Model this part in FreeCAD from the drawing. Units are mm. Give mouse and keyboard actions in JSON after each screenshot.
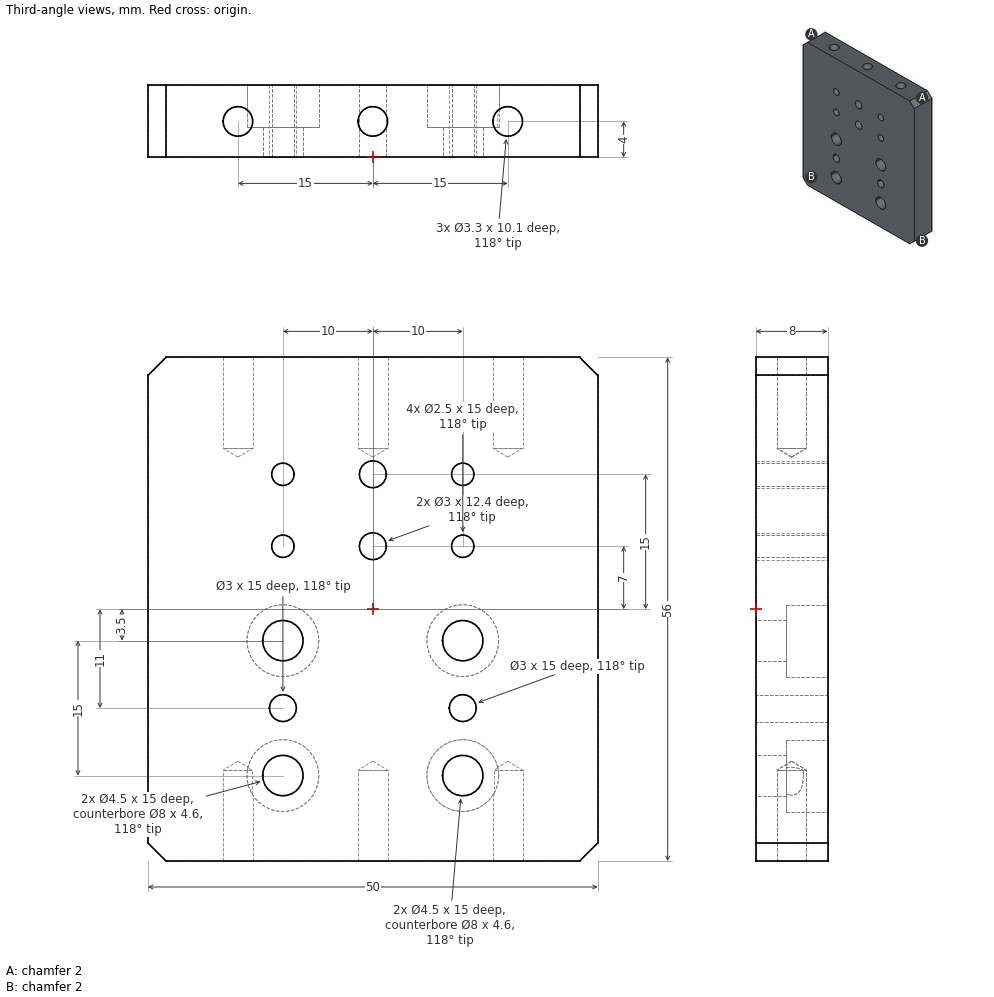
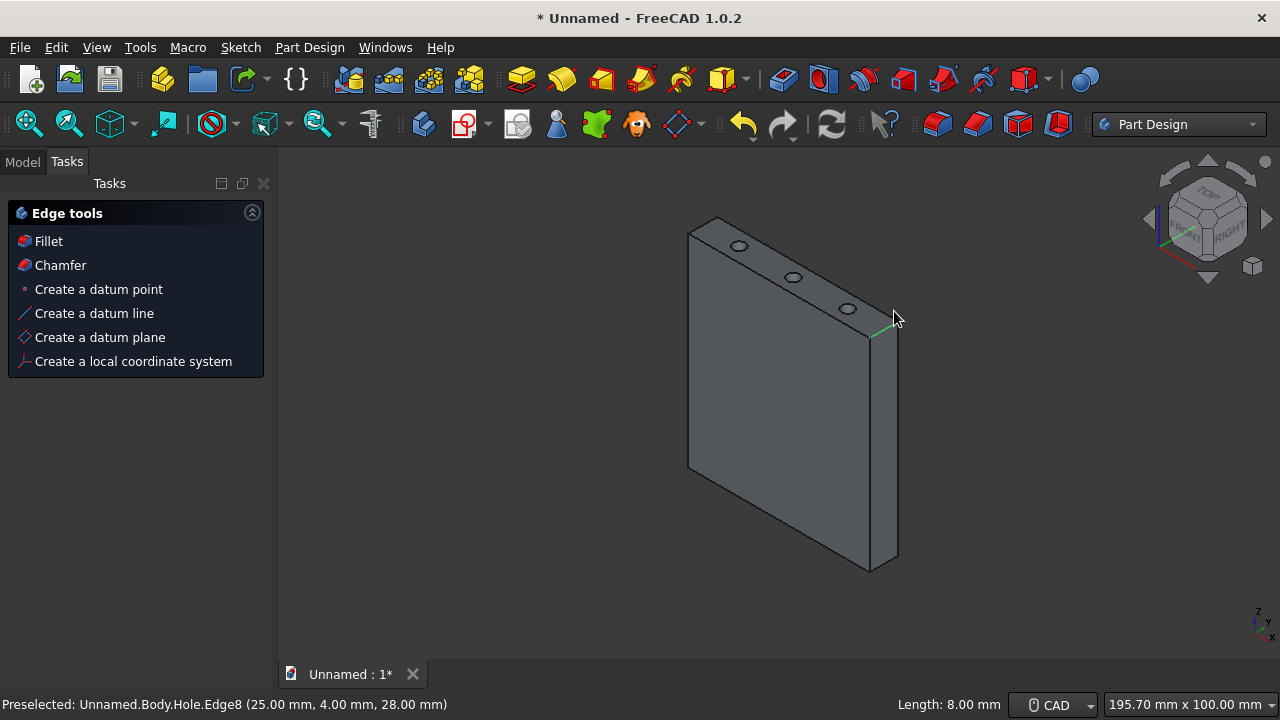
{"action": "key", "text": "2"}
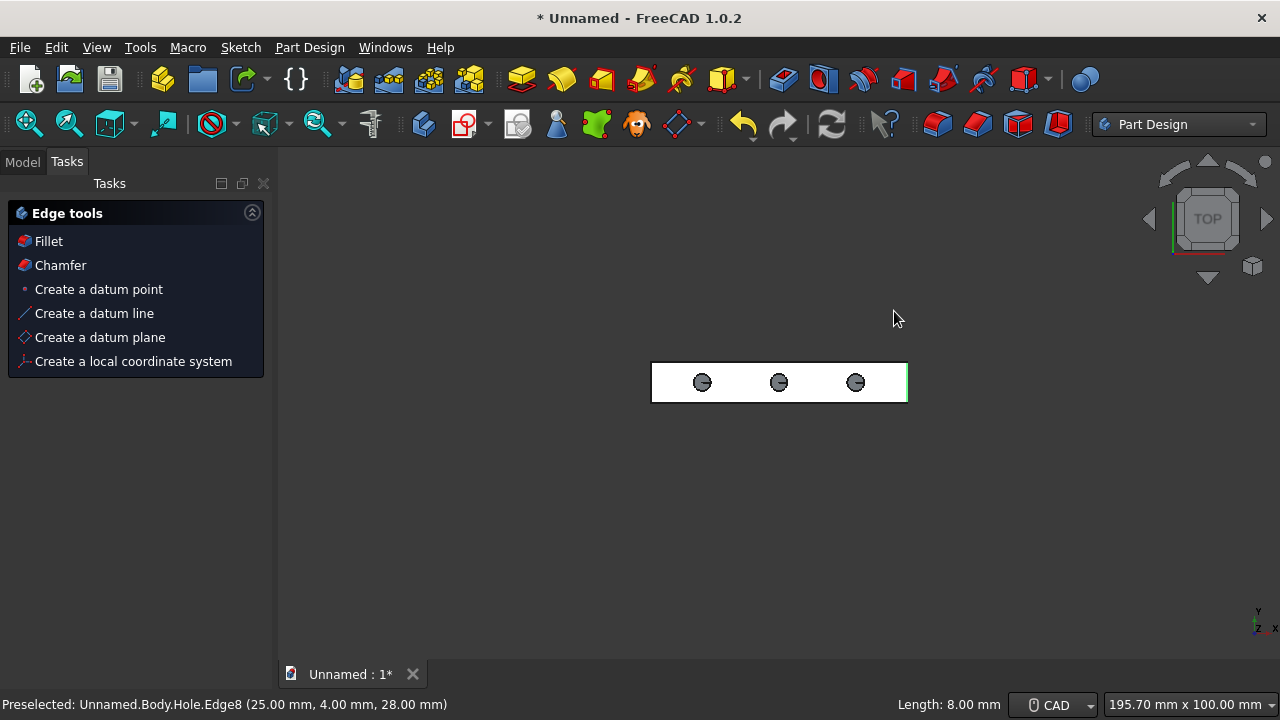
{"action": "left_click", "coordinate": [30, 124]}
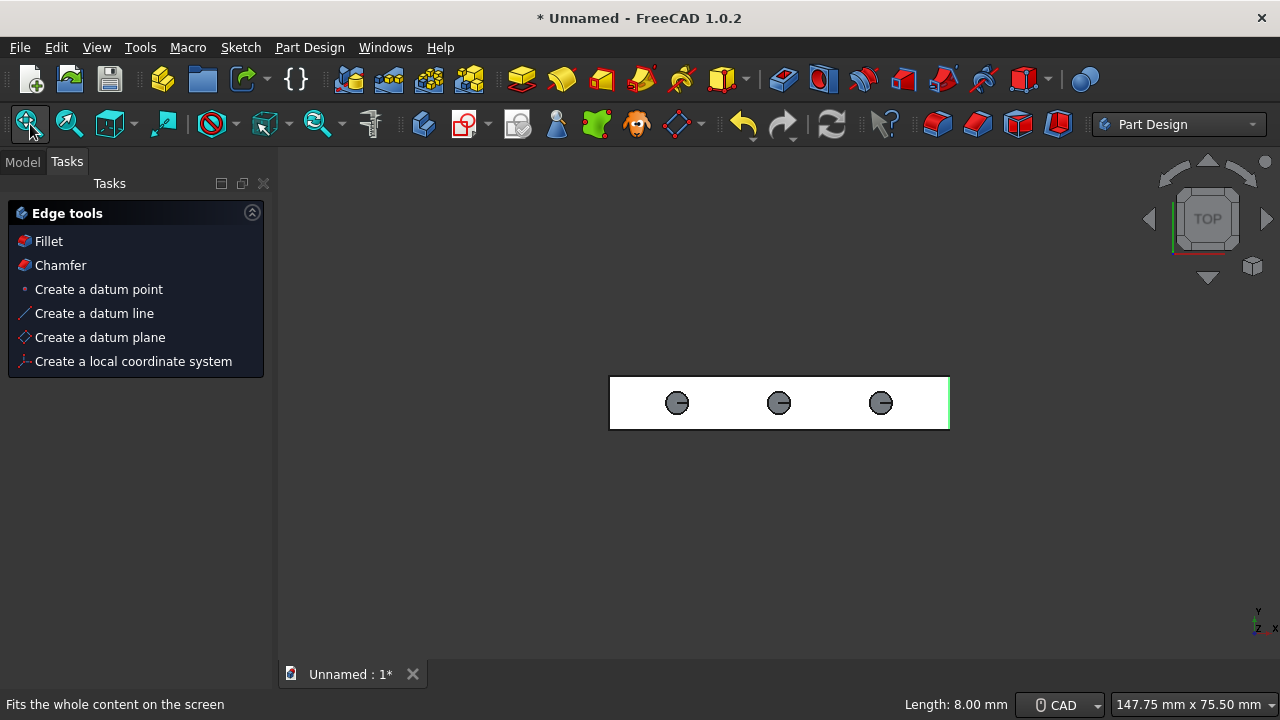
{"action": "left_click", "coordinate": [609, 402], "text": "ctrl"}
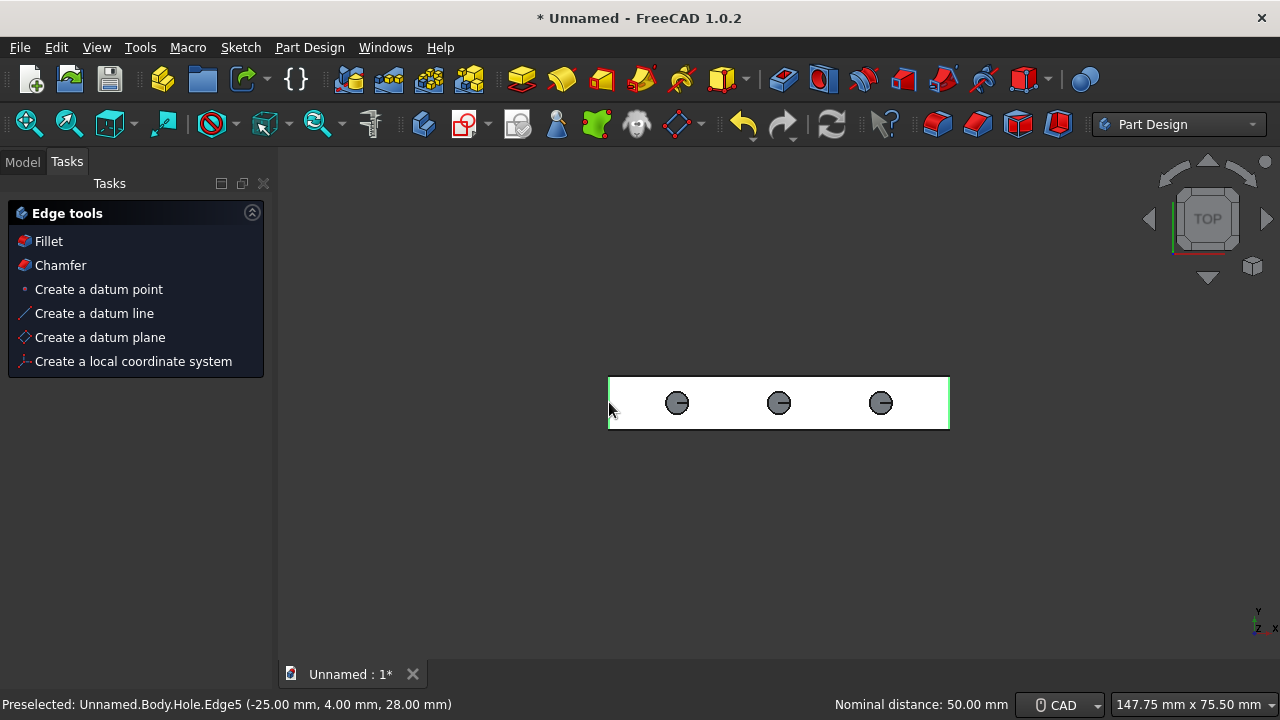
{"action": "left_click", "coordinate": [978, 124]}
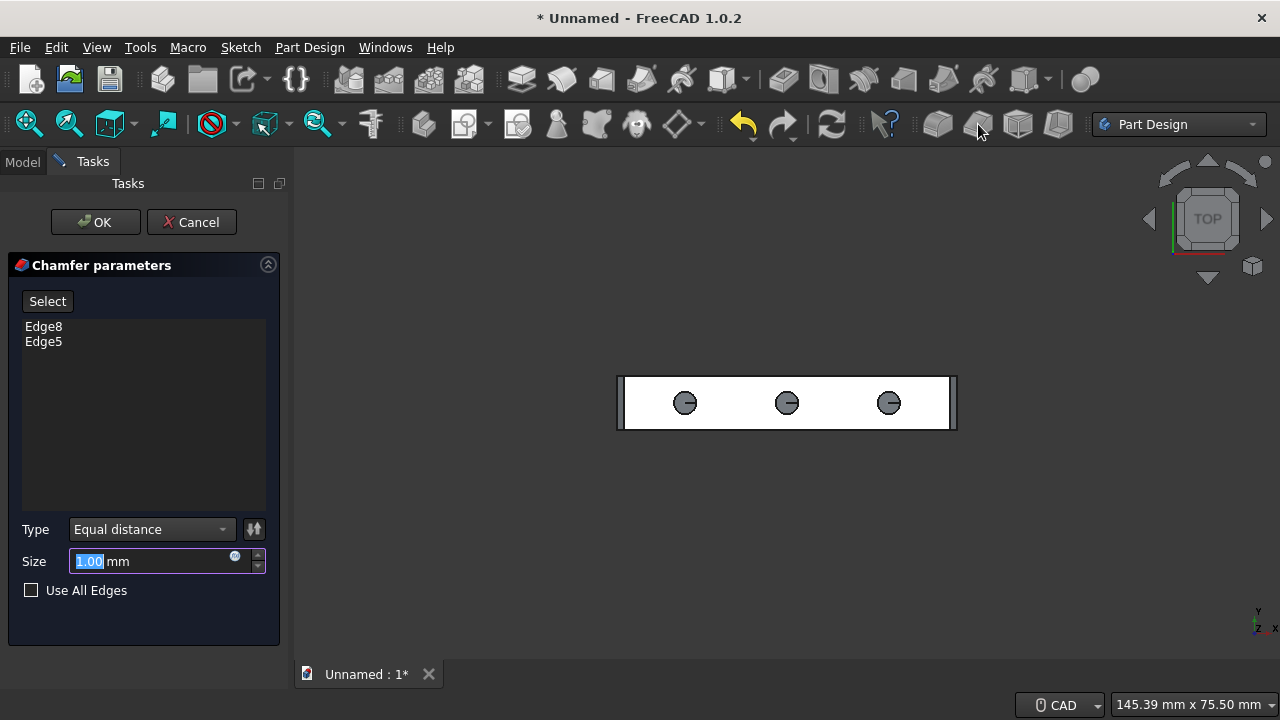
{"action": "type", "text": "2"}
{"action": "key", "text": "Tab"}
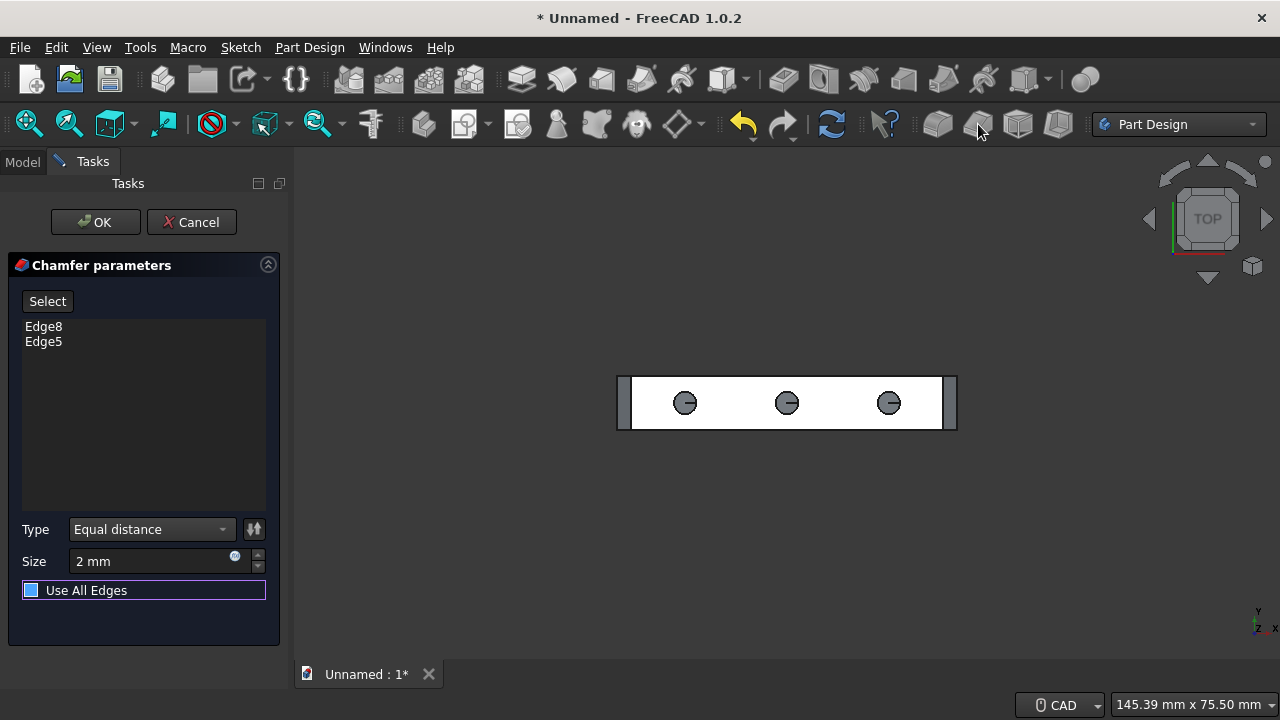
{"action": "left_click", "coordinate": [96, 222]}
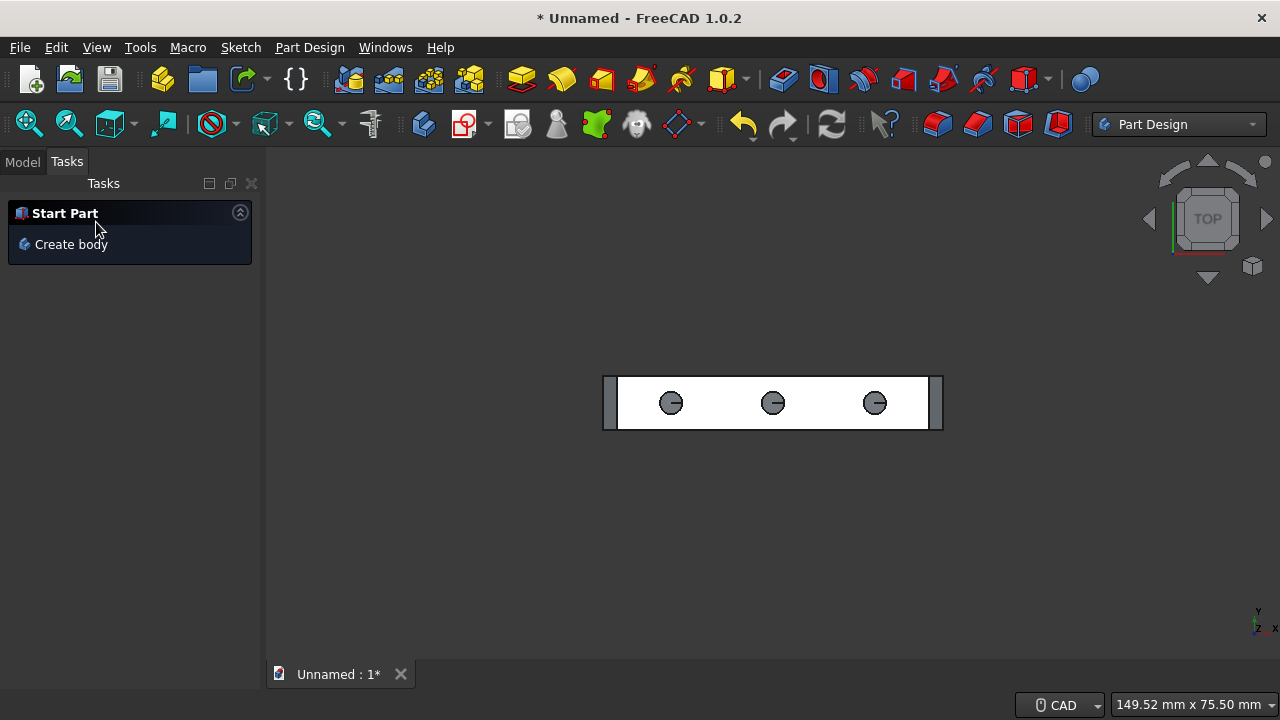
{"action": "left_click", "coordinate": [30, 124]}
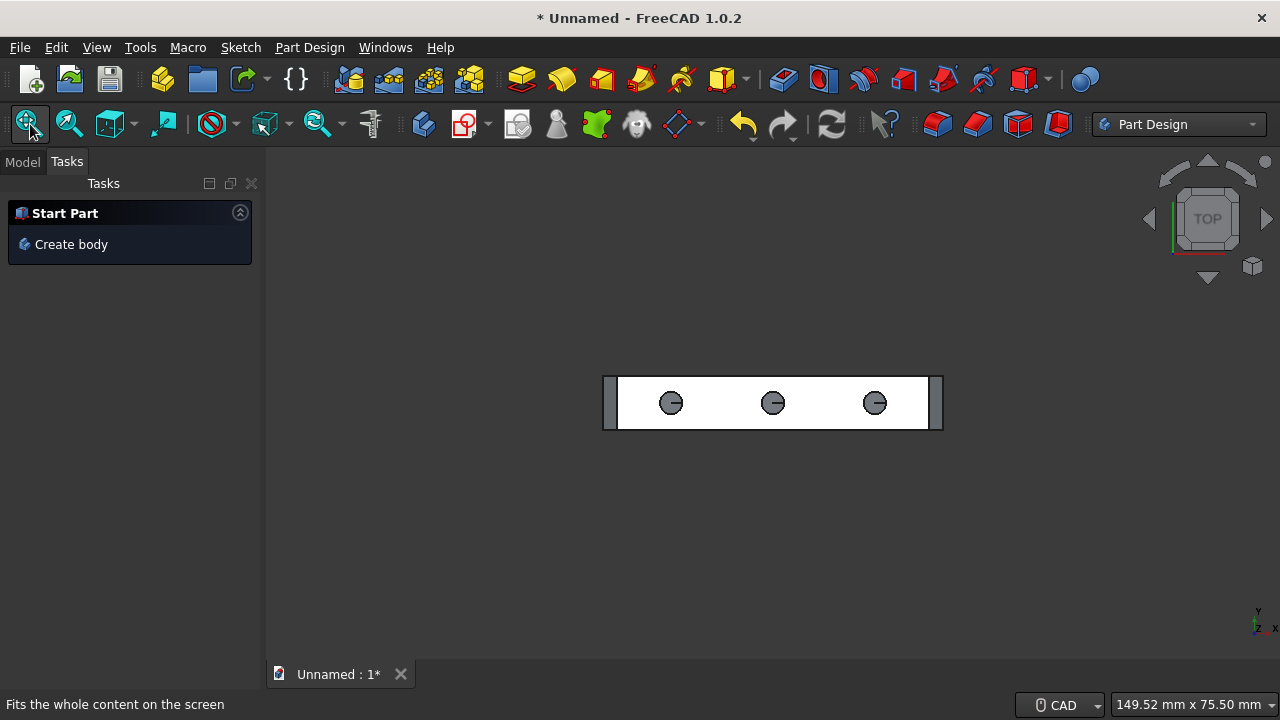
{"action": "key", "text": "5"}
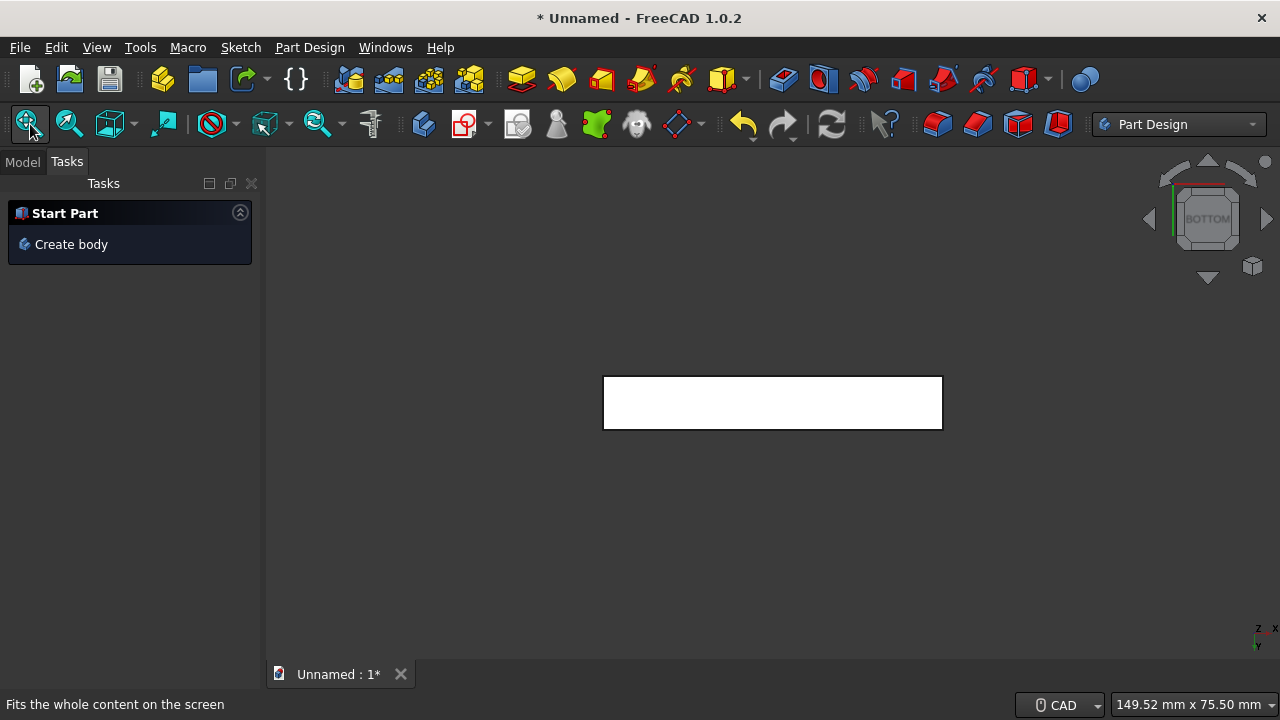
{"action": "left_click", "coordinate": [30, 124]}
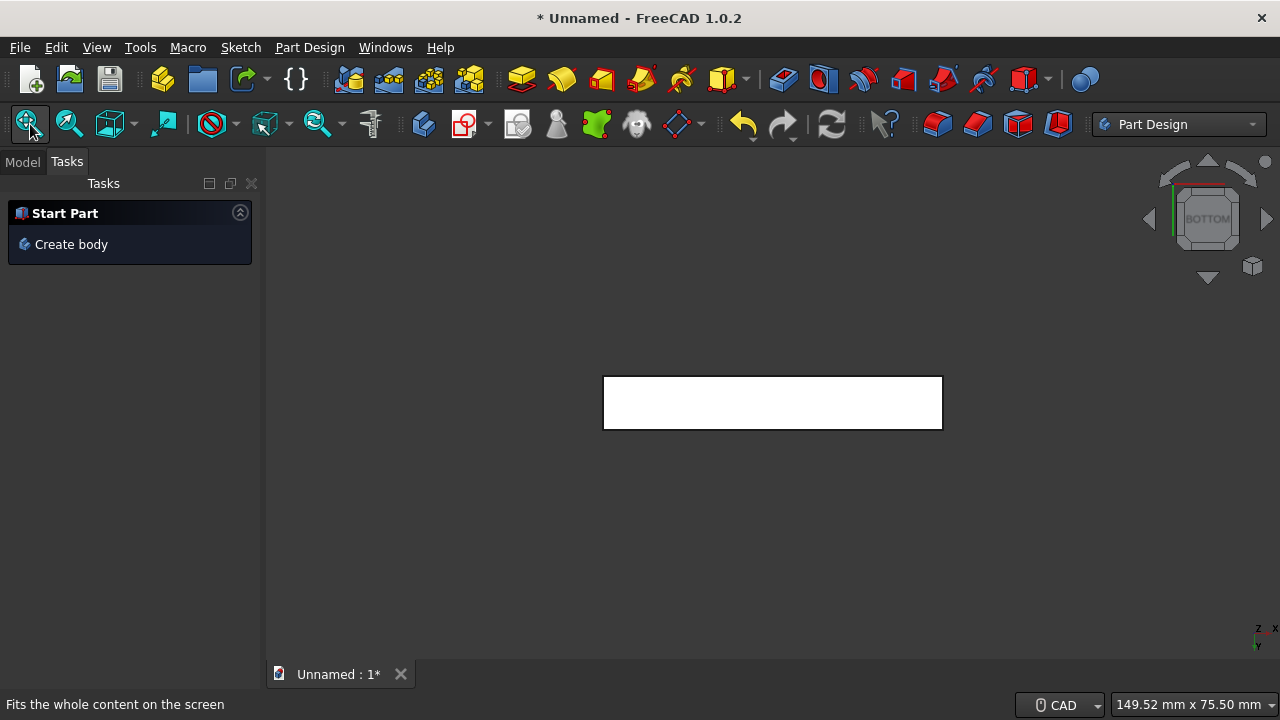
{"action": "left_click", "coordinate": [870, 402]}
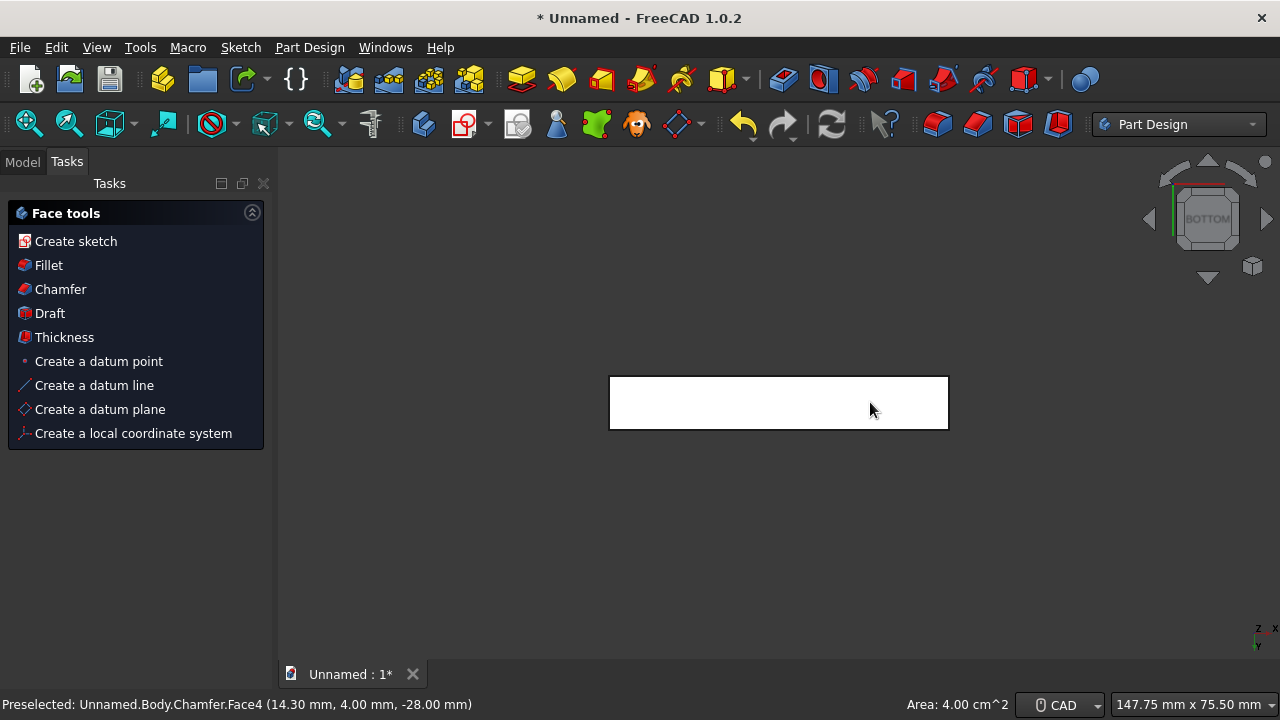
{"action": "left_click", "coordinate": [464, 124]}